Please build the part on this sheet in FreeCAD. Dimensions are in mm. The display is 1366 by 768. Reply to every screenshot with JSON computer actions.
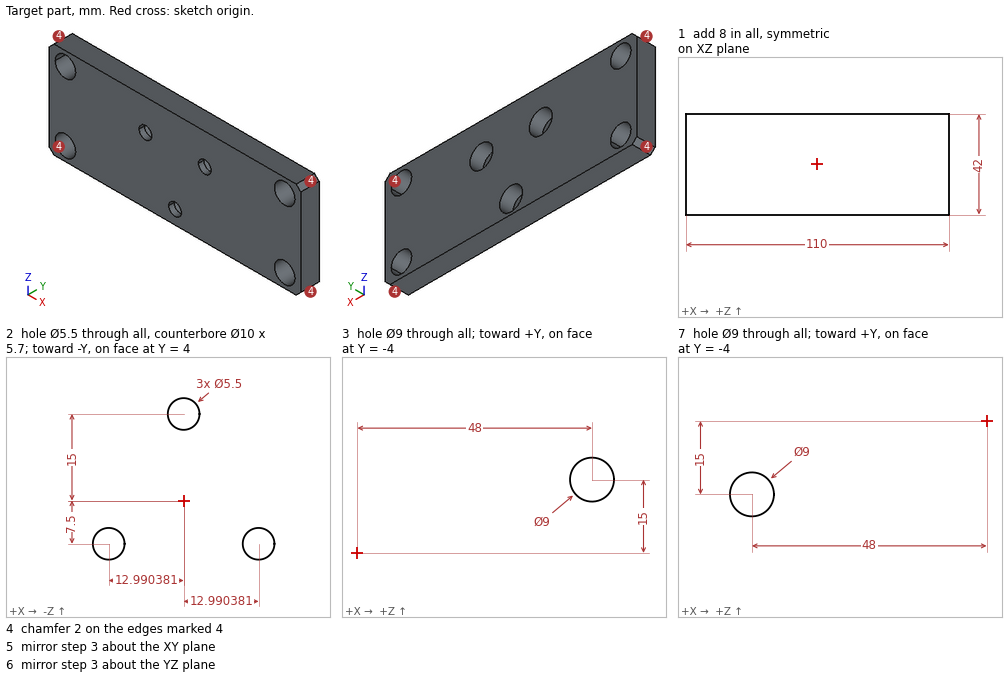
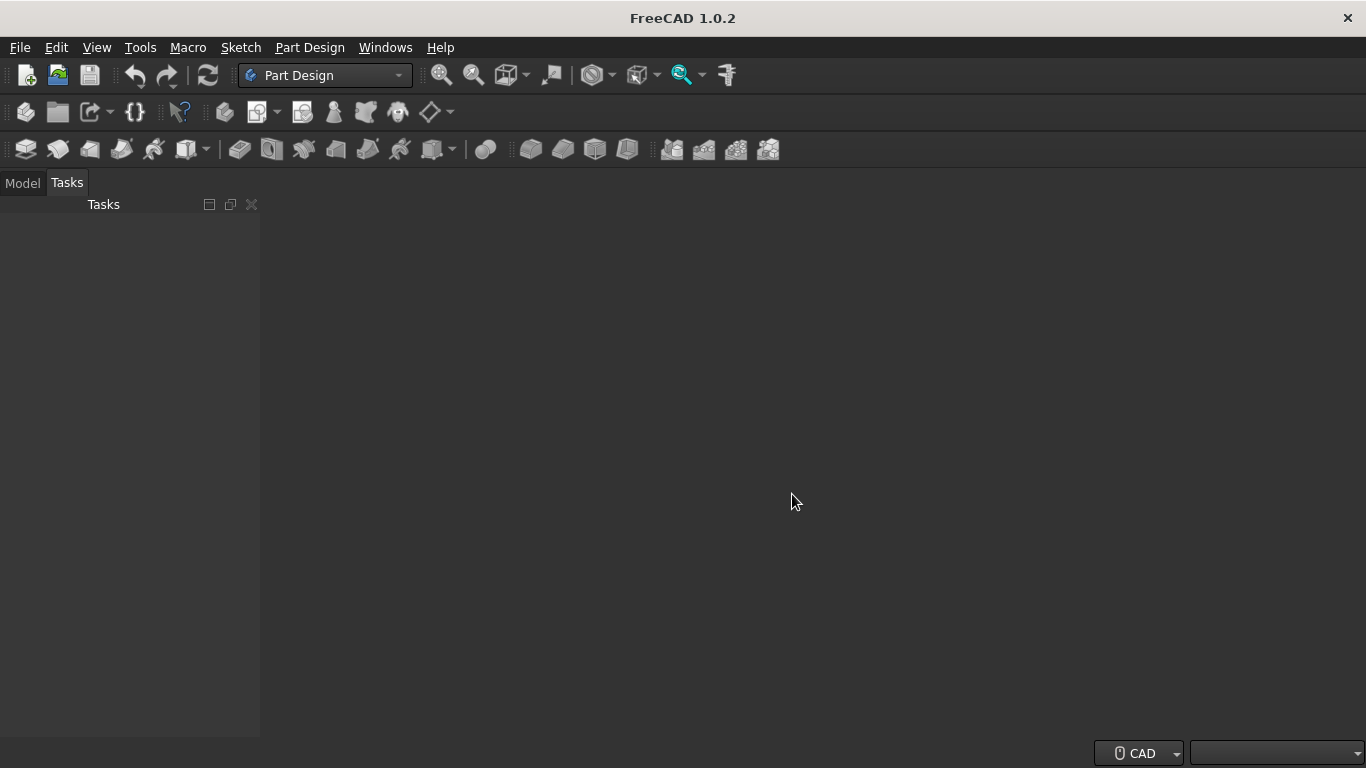
{"action": "left_click", "coordinate": [26, 76]}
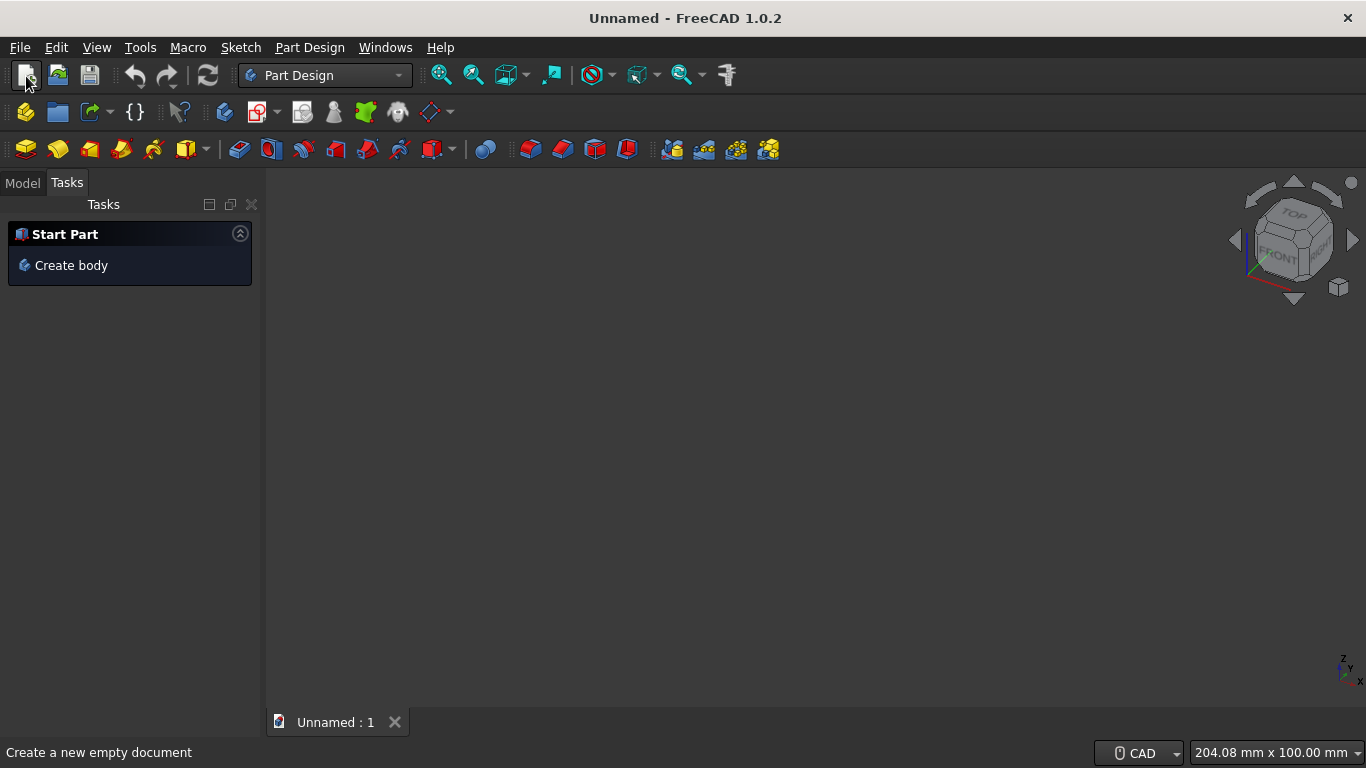
{"action": "left_click", "coordinate": [258, 112]}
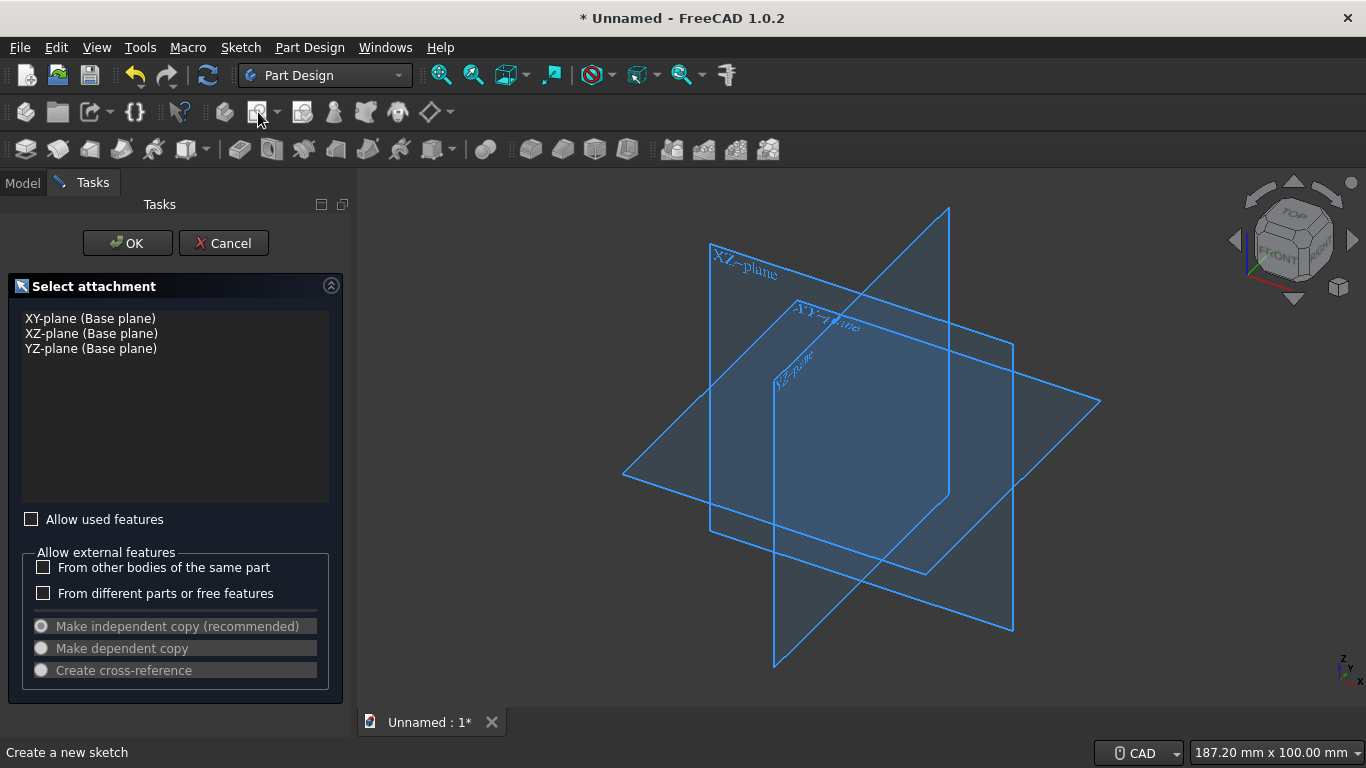
{"action": "left_click", "coordinate": [82, 334]}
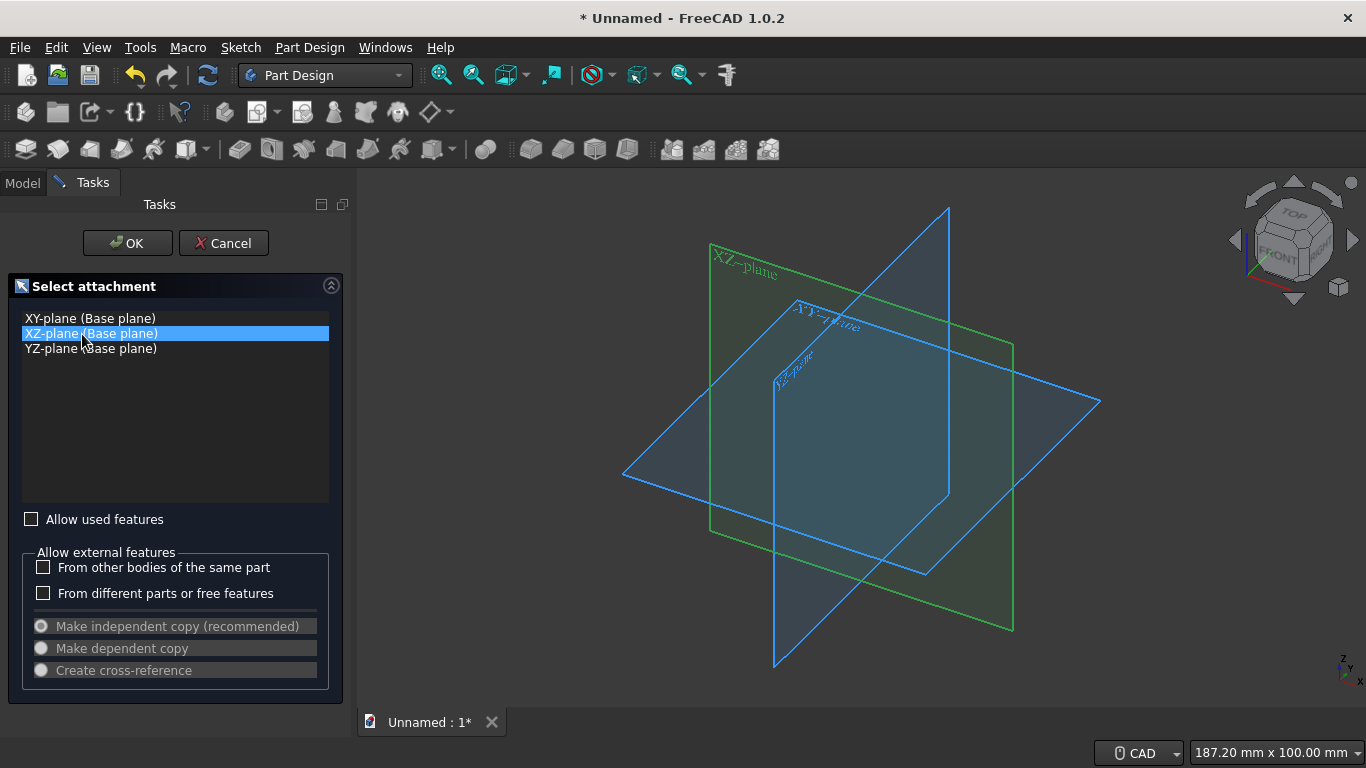
{"action": "left_click", "coordinate": [128, 243]}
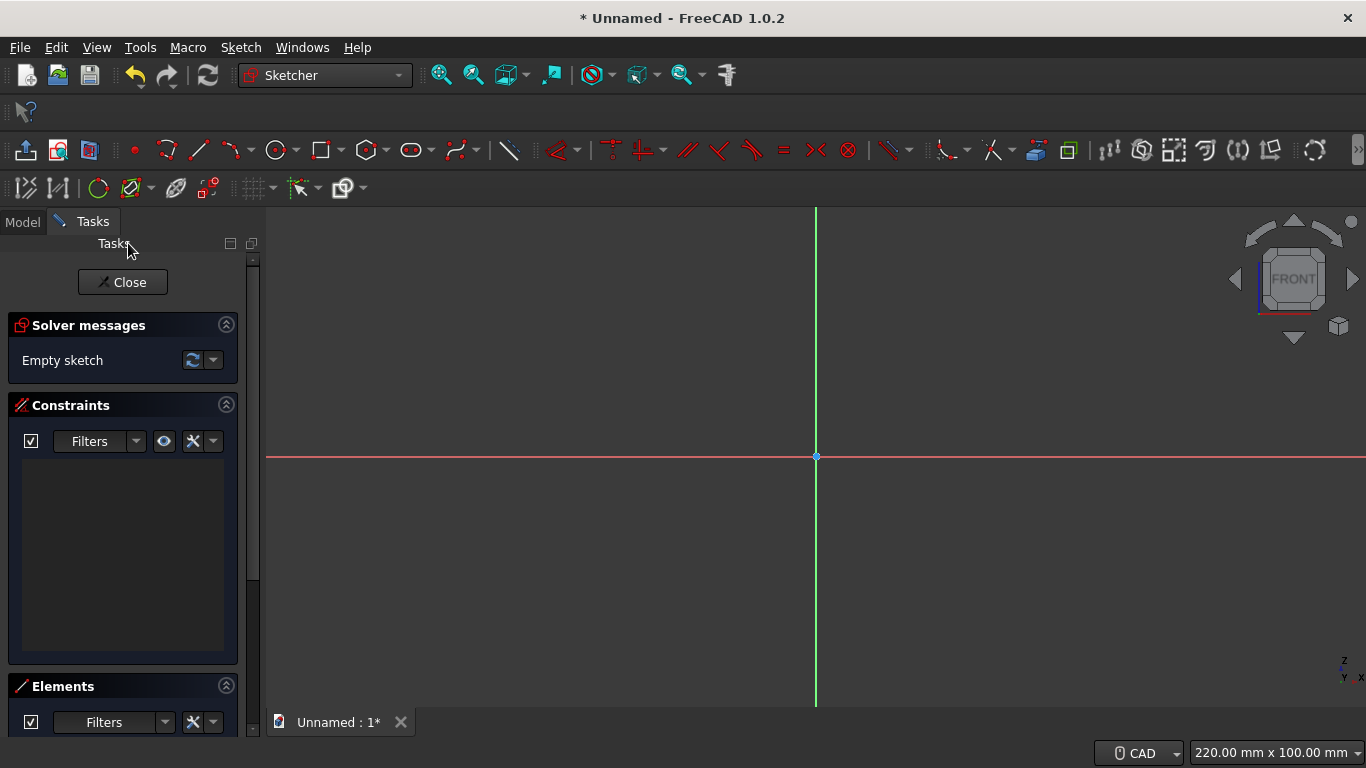
{"action": "key", "text": "g v"}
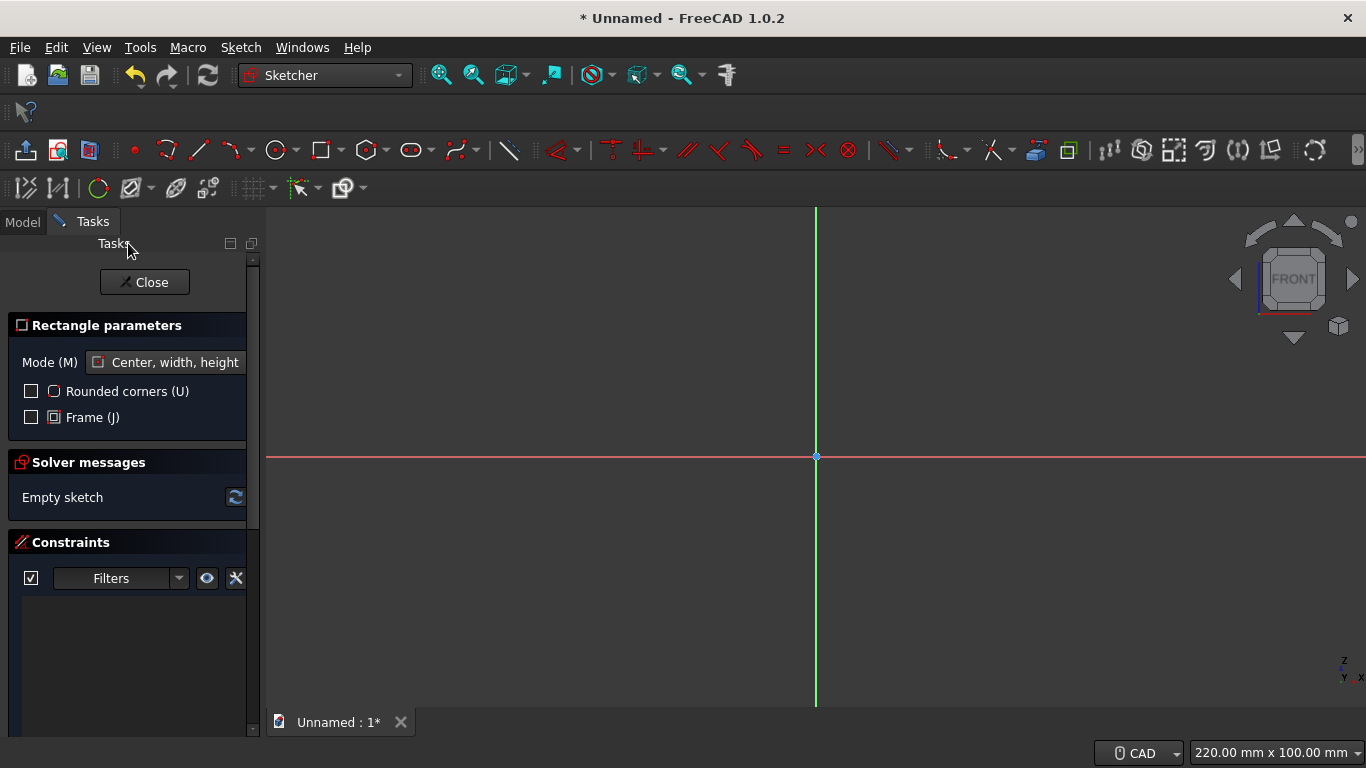
{"action": "left_click", "coordinate": [816, 457]}
{"action": "left_click", "coordinate": [1091, 352]}
{"action": "key", "text": "Escape"}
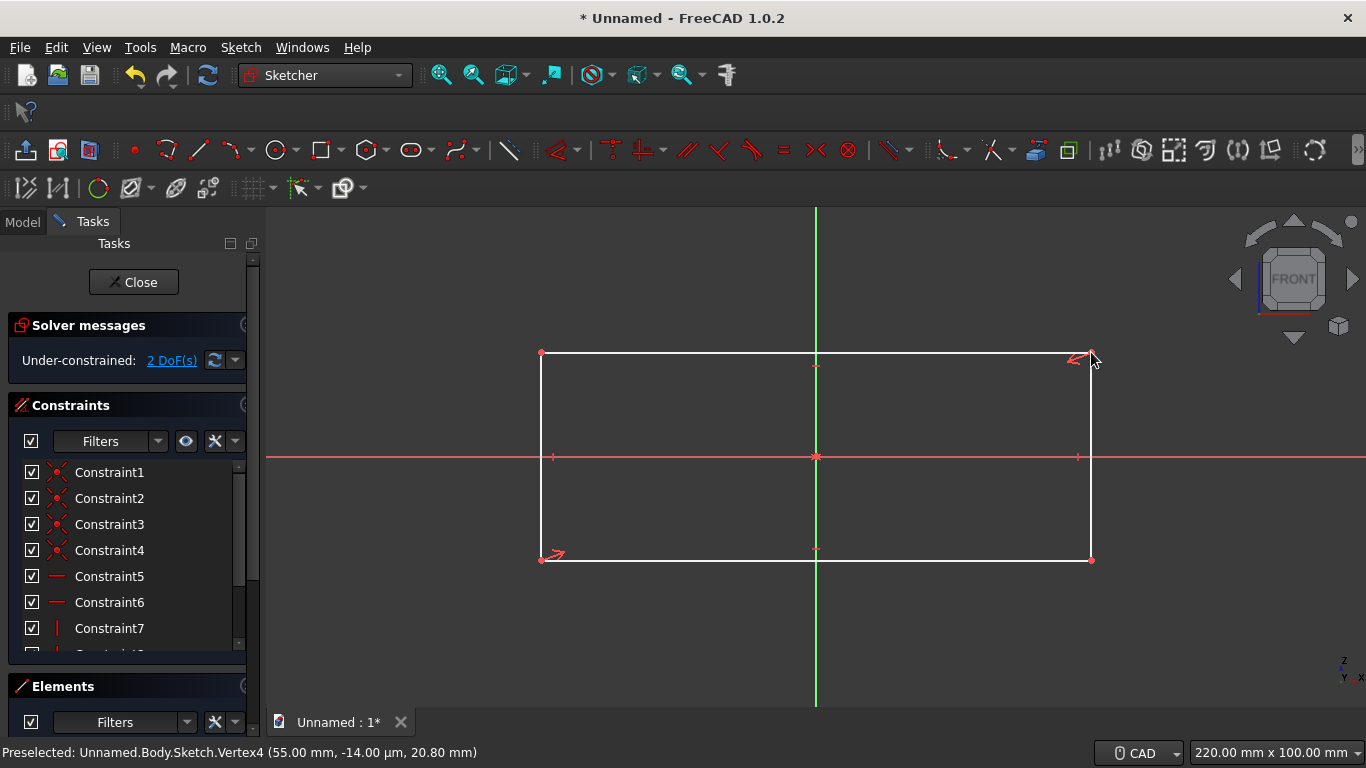
{"action": "left_click", "coordinate": [556, 150]}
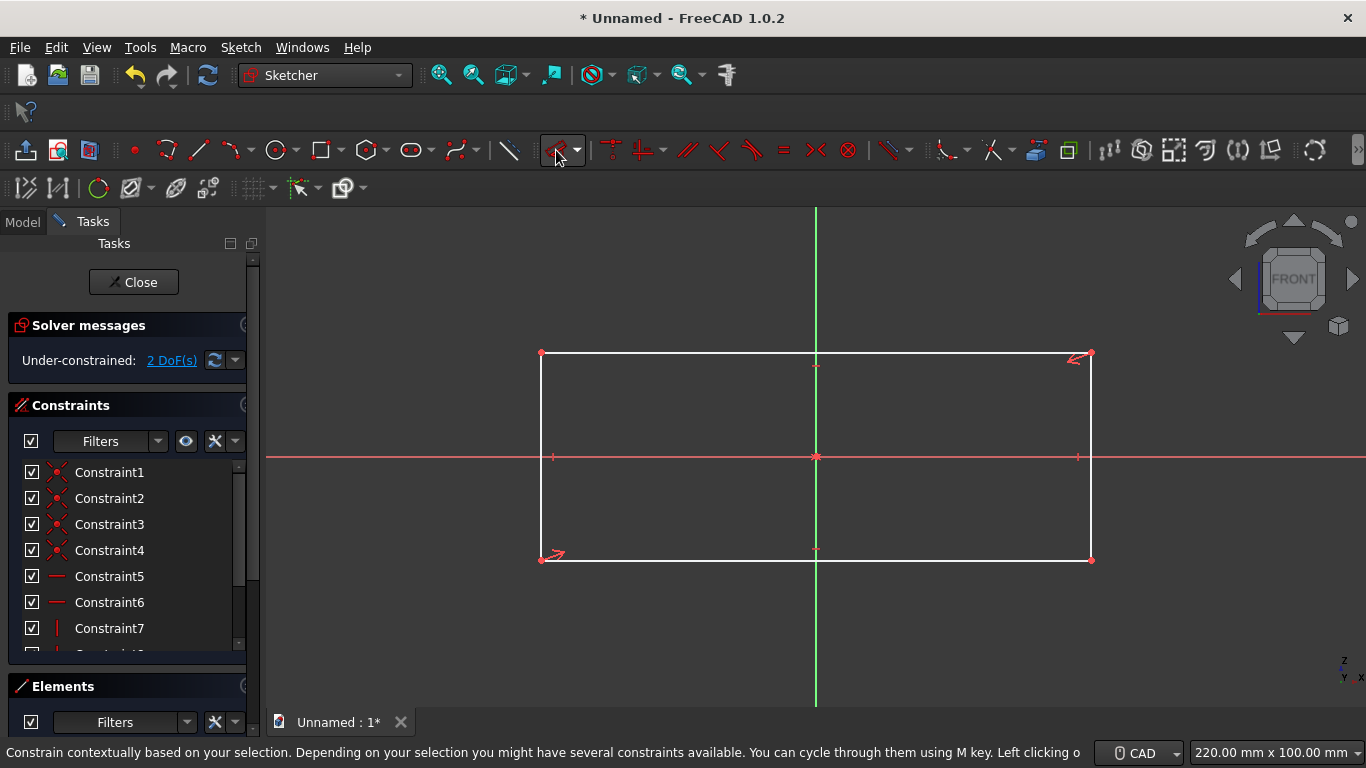
{"action": "left_click", "coordinate": [1091, 499]}
{"action": "left_click", "coordinate": [1125, 409]}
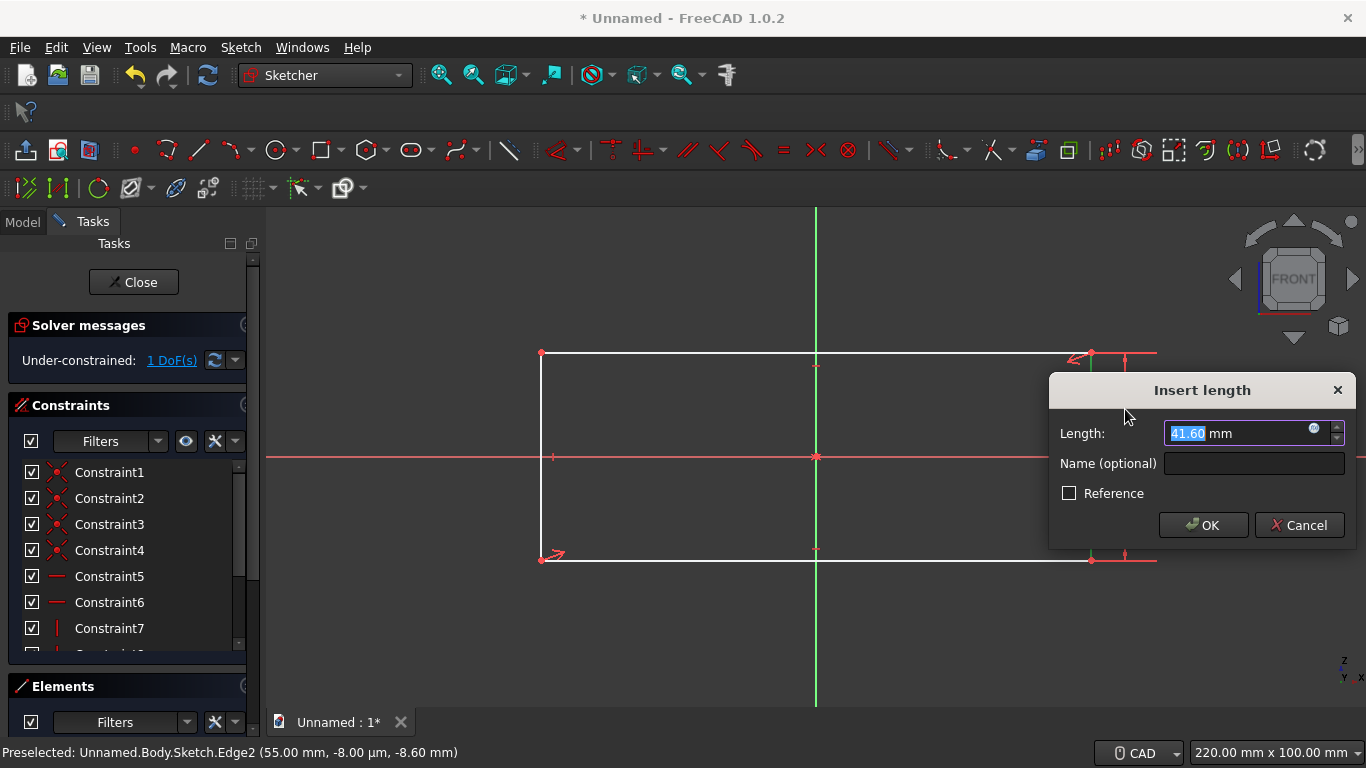
{"action": "type", "text": "42"}
{"action": "key", "text": "Return"}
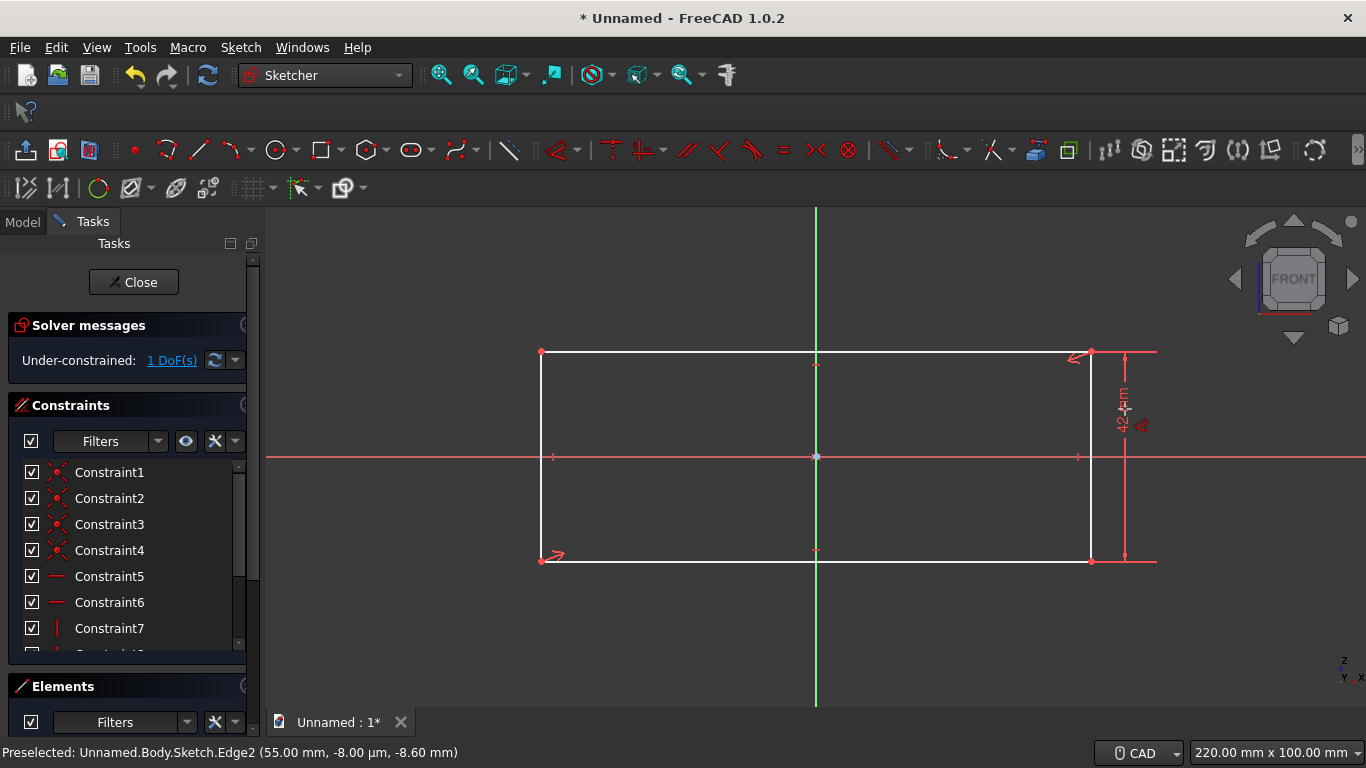
{"action": "left_click", "coordinate": [706, 562]}
{"action": "left_click", "coordinate": [690, 596]}